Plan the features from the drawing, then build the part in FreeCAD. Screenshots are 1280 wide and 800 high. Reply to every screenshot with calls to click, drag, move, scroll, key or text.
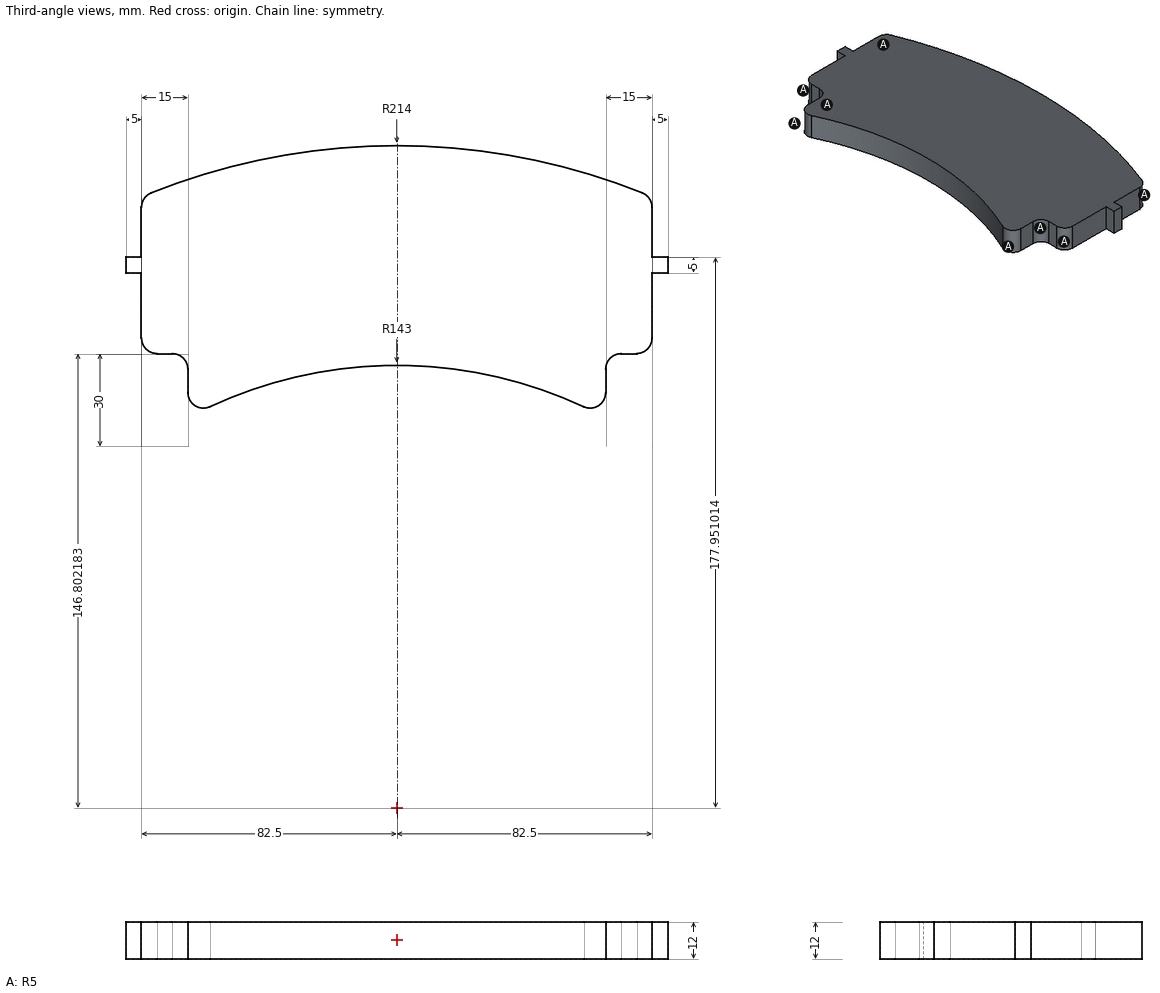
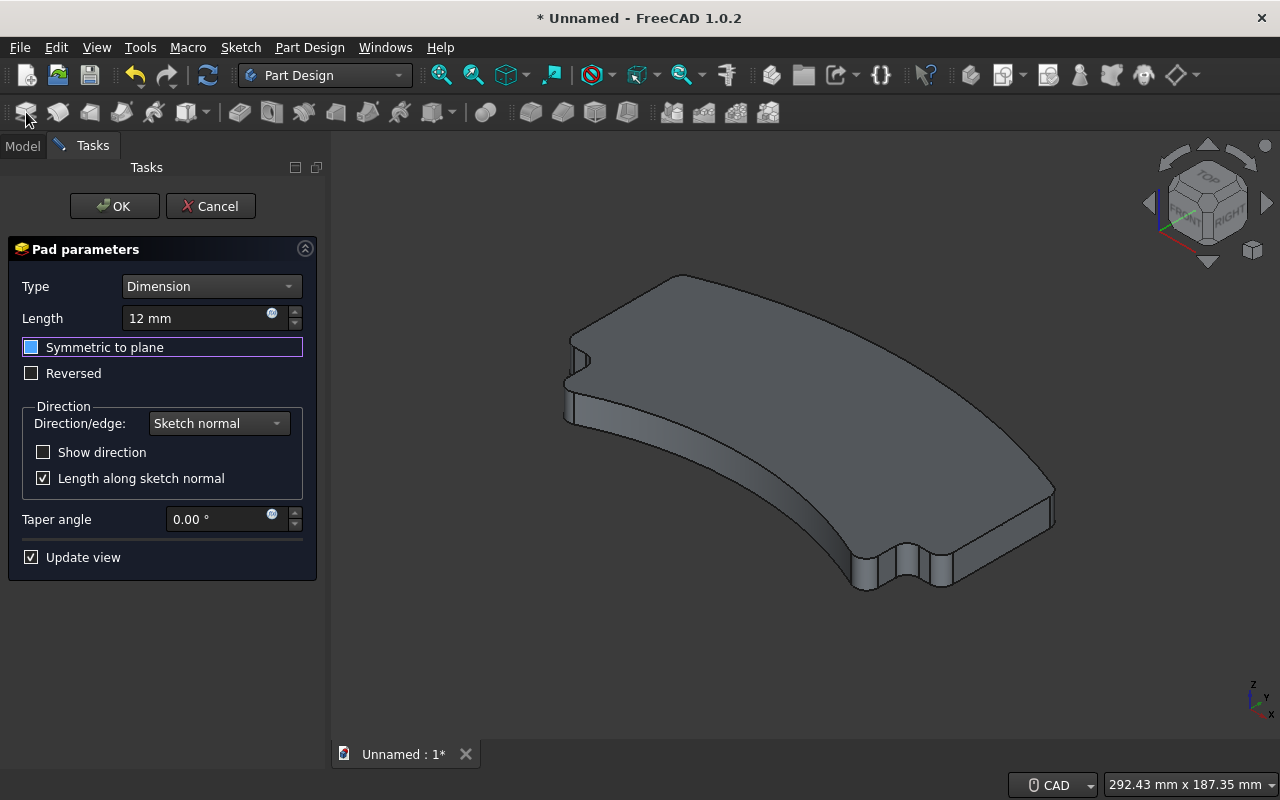
click(30, 373)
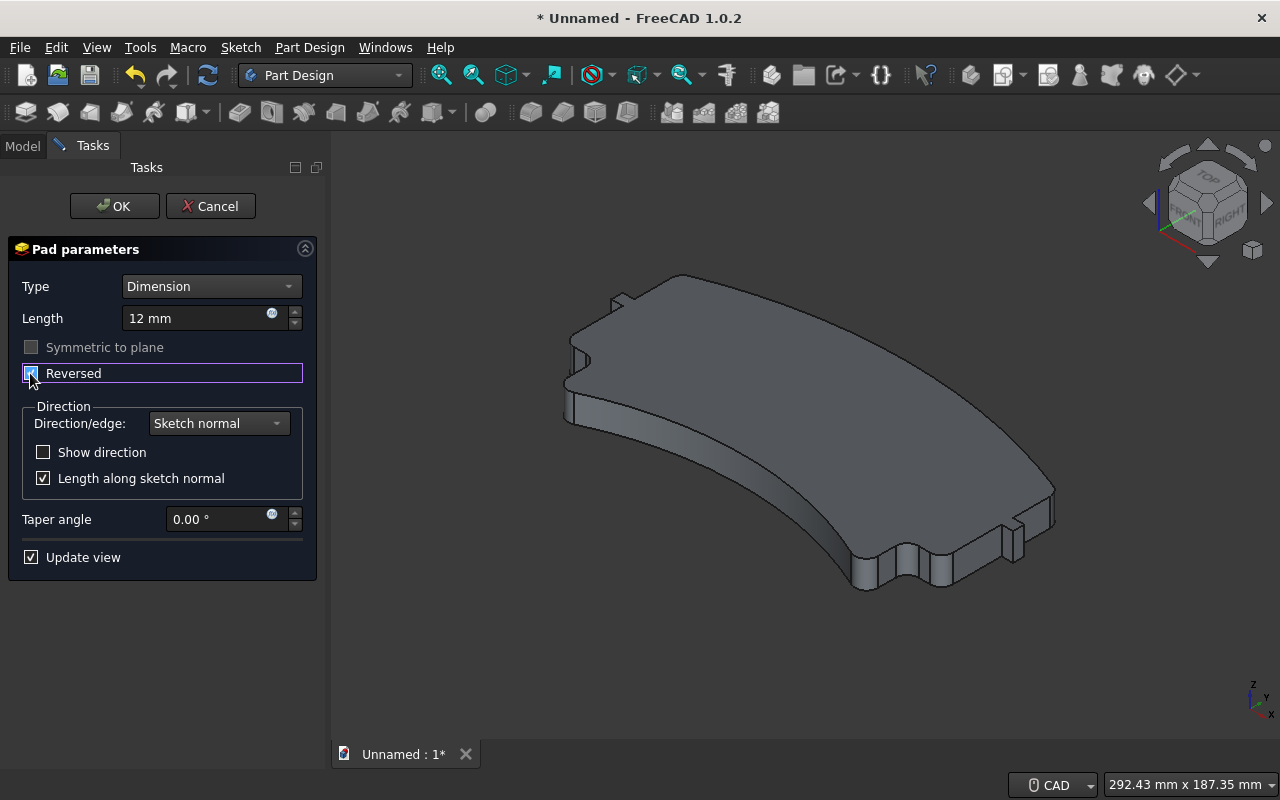
click(115, 206)